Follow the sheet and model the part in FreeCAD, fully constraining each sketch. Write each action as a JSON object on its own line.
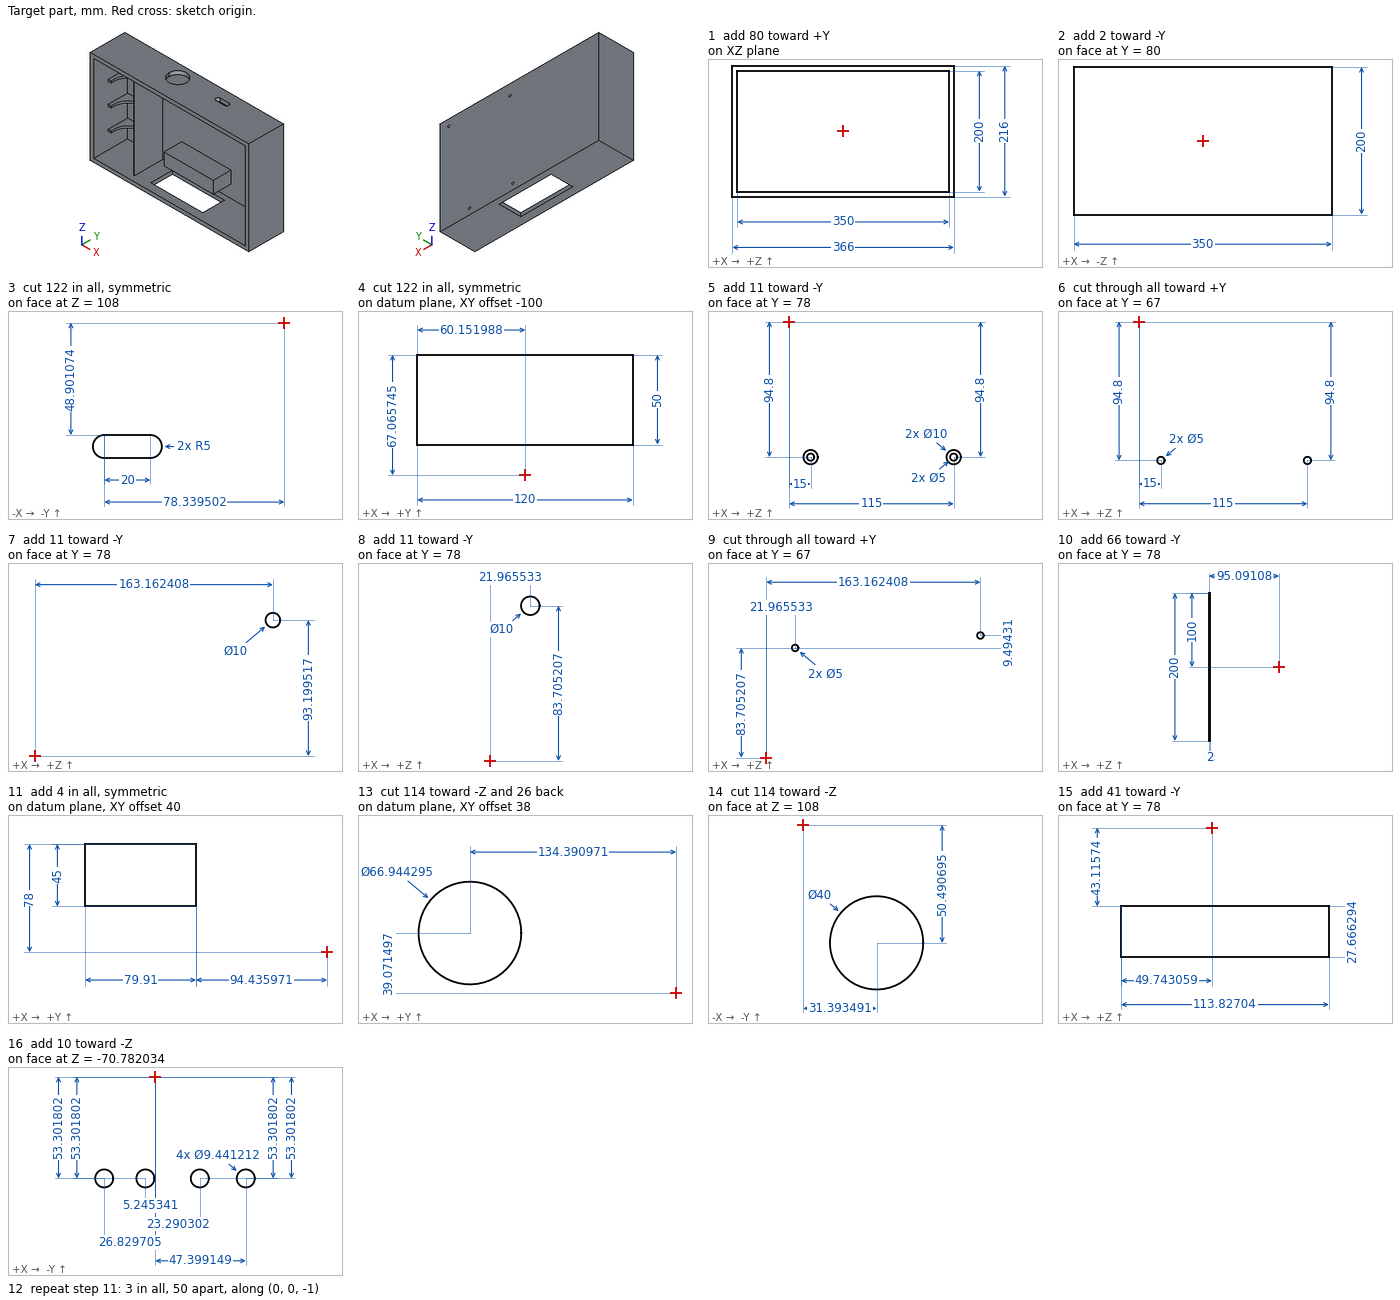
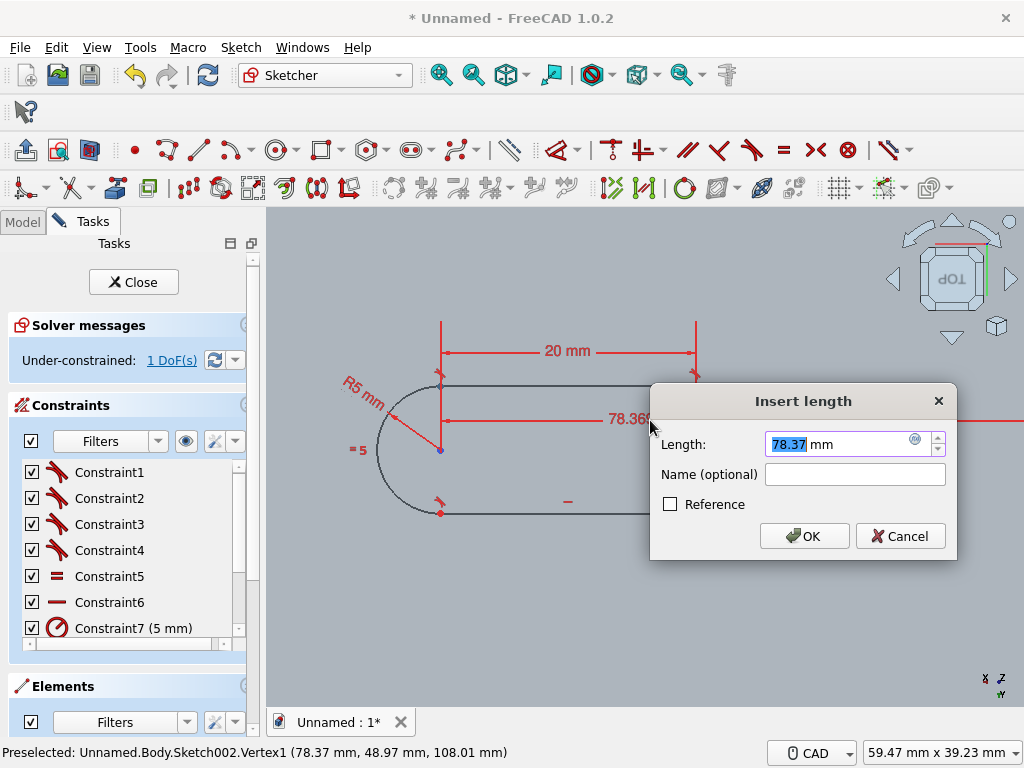
{"action": "type", "text": "78.339502"}
{"action": "key", "text": "Return"}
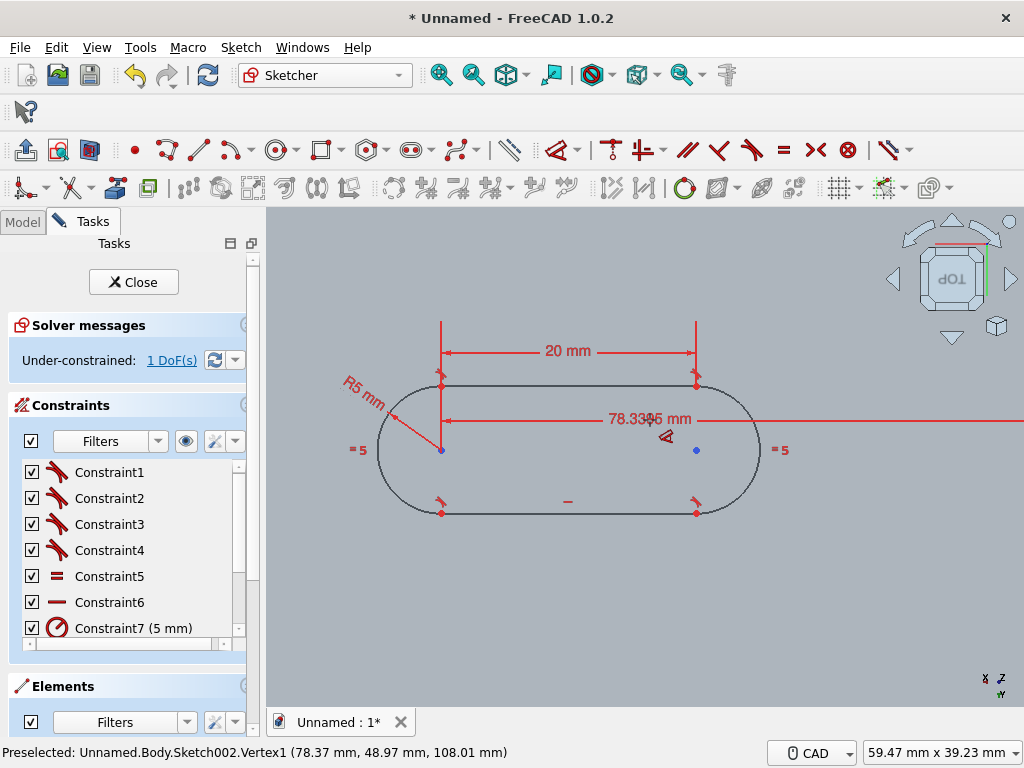
{"action": "left_click", "coordinate": [441, 386]}
{"action": "left_click", "coordinate": [407, 311]}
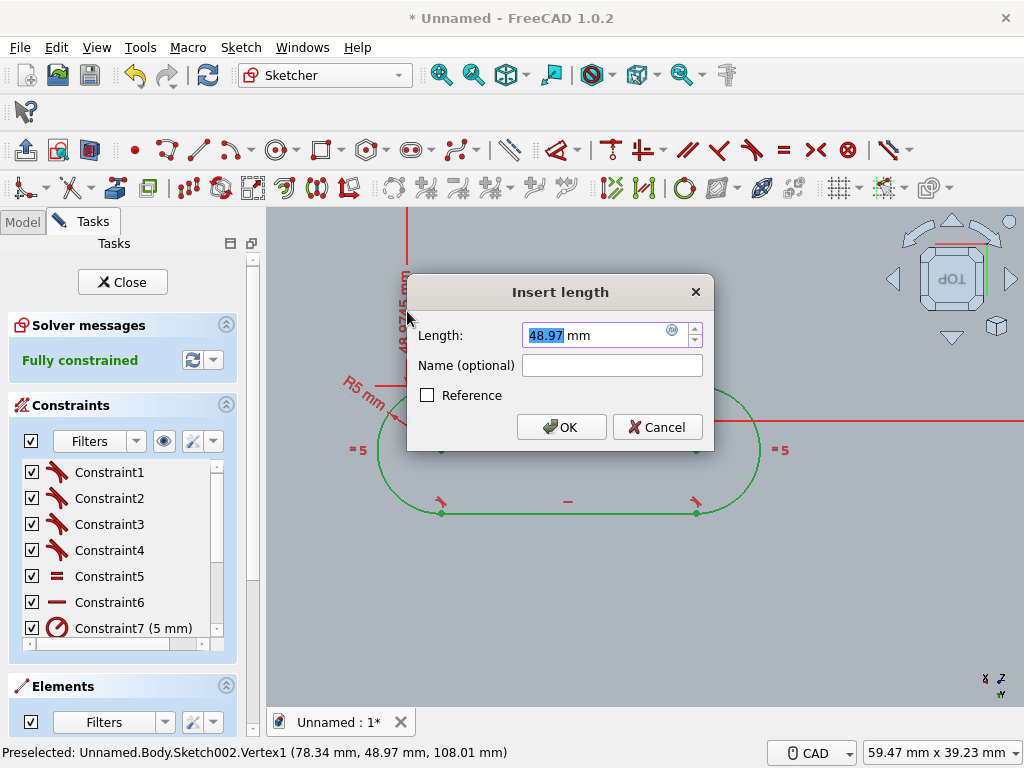
{"action": "type", "text": "48.901074"}
{"action": "key", "text": "Return"}
{"action": "key", "text": "Escape"}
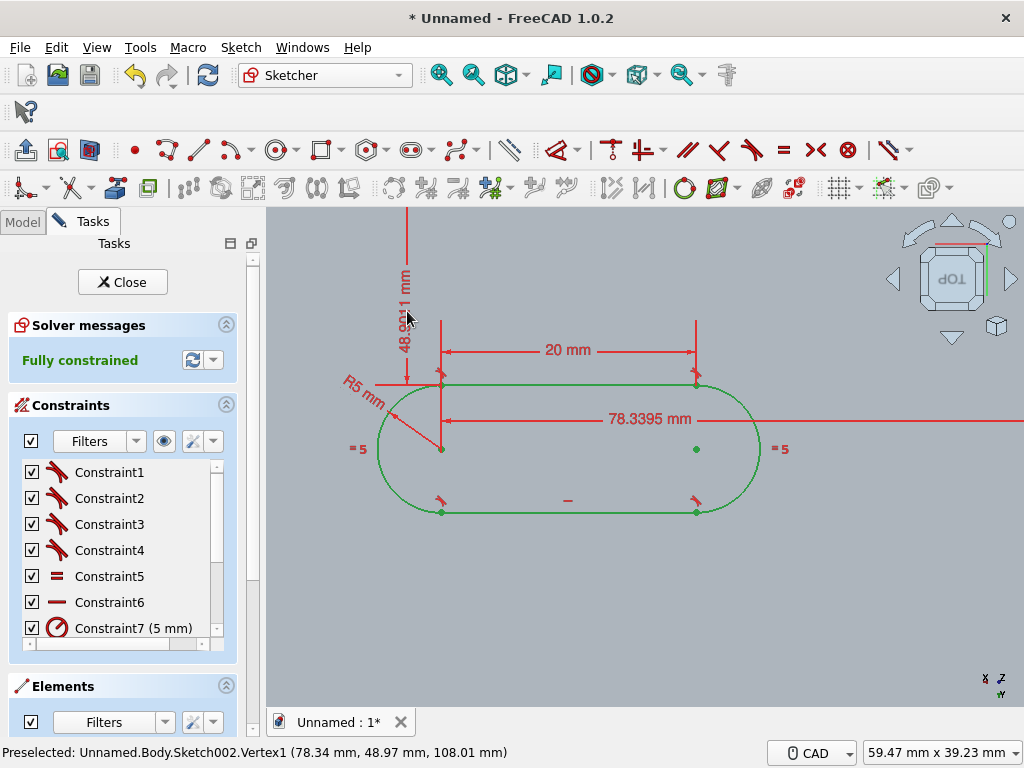
{"action": "left_click", "coordinate": [123, 282]}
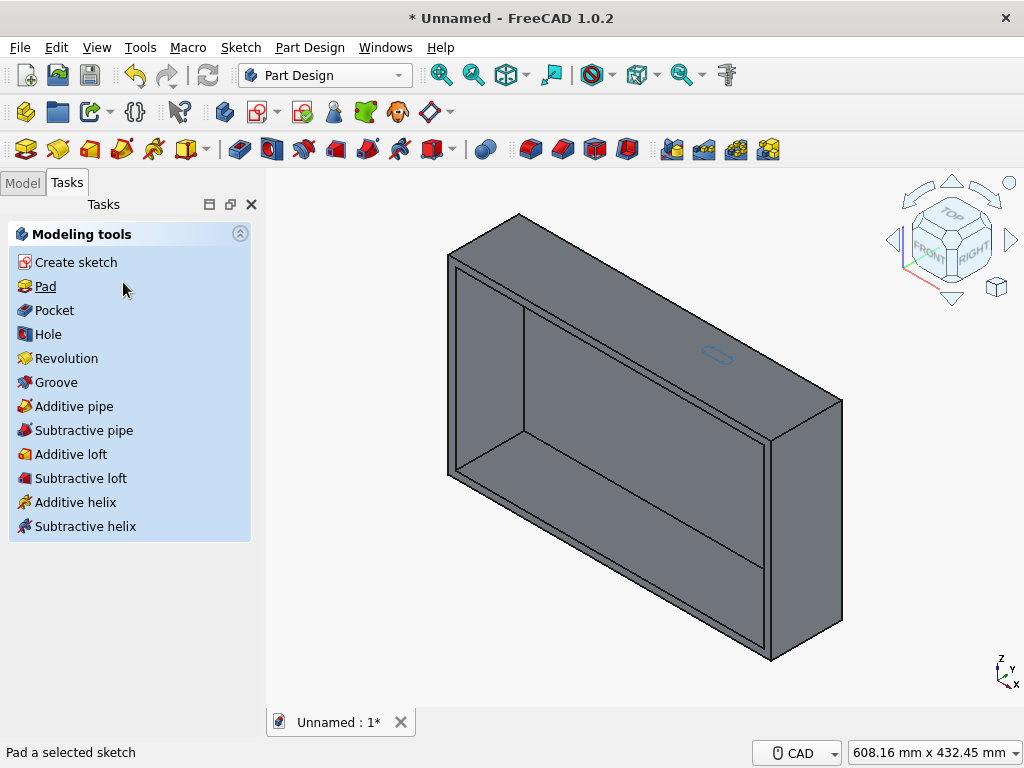
{"action": "left_click", "coordinate": [240, 150]}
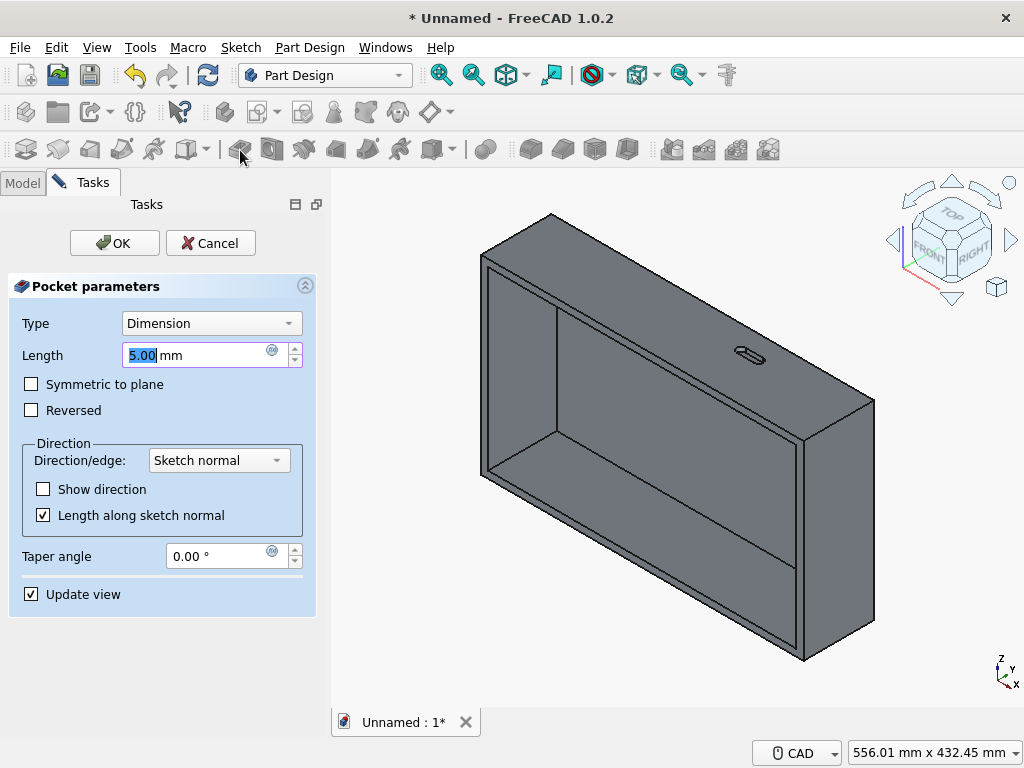
{"action": "type", "text": "122"}
{"action": "key", "text": "Tab"}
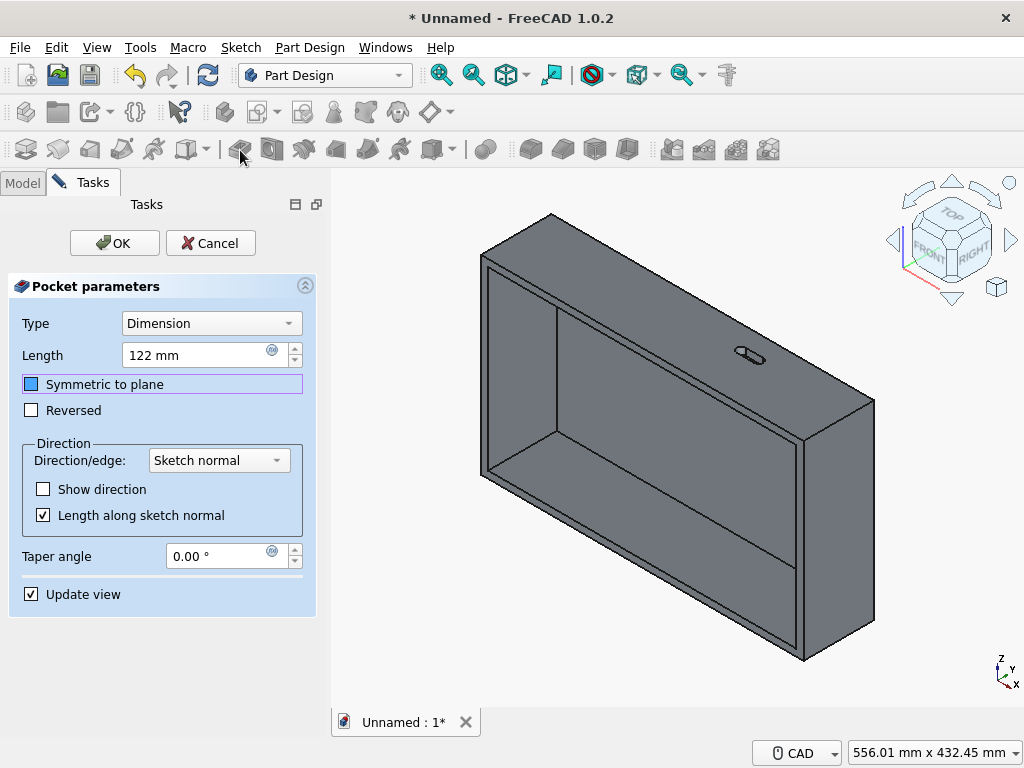
{"action": "left_click", "coordinate": [30, 384]}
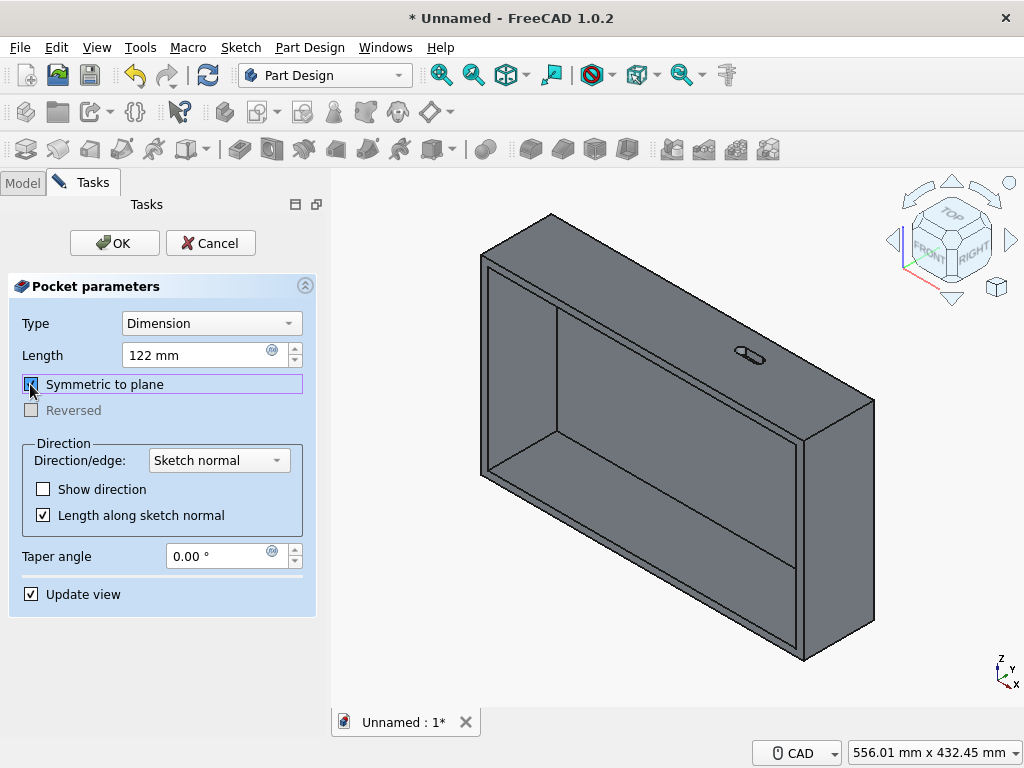
{"action": "left_click", "coordinate": [115, 243]}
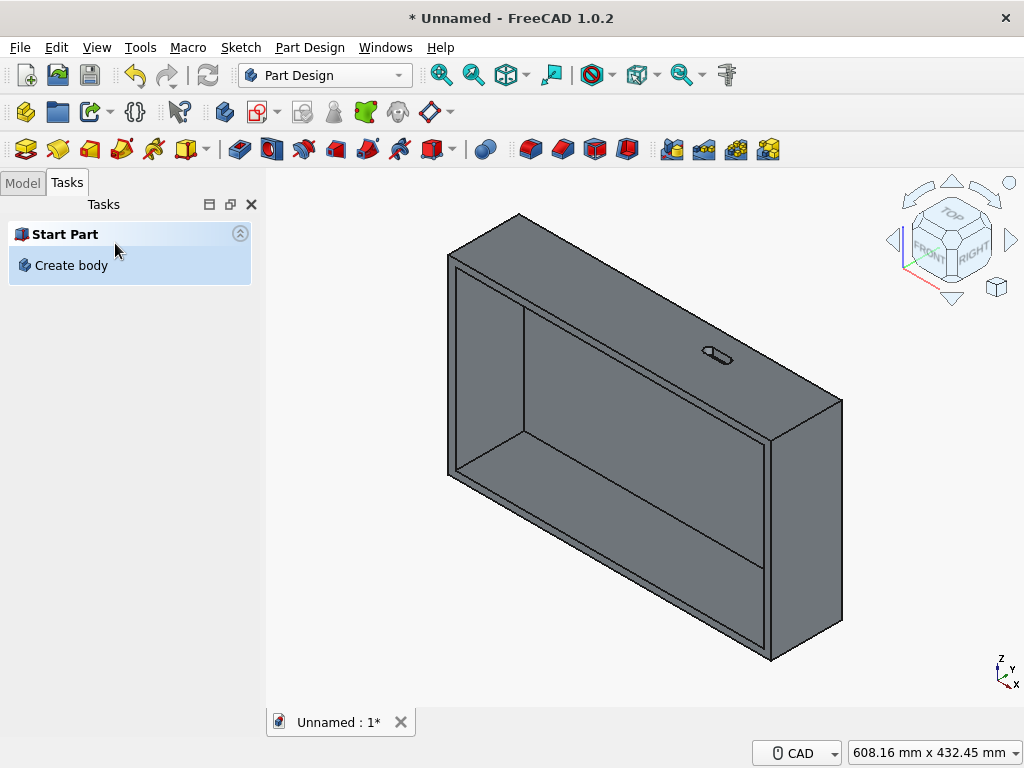
{"action": "left_click", "coordinate": [23, 182]}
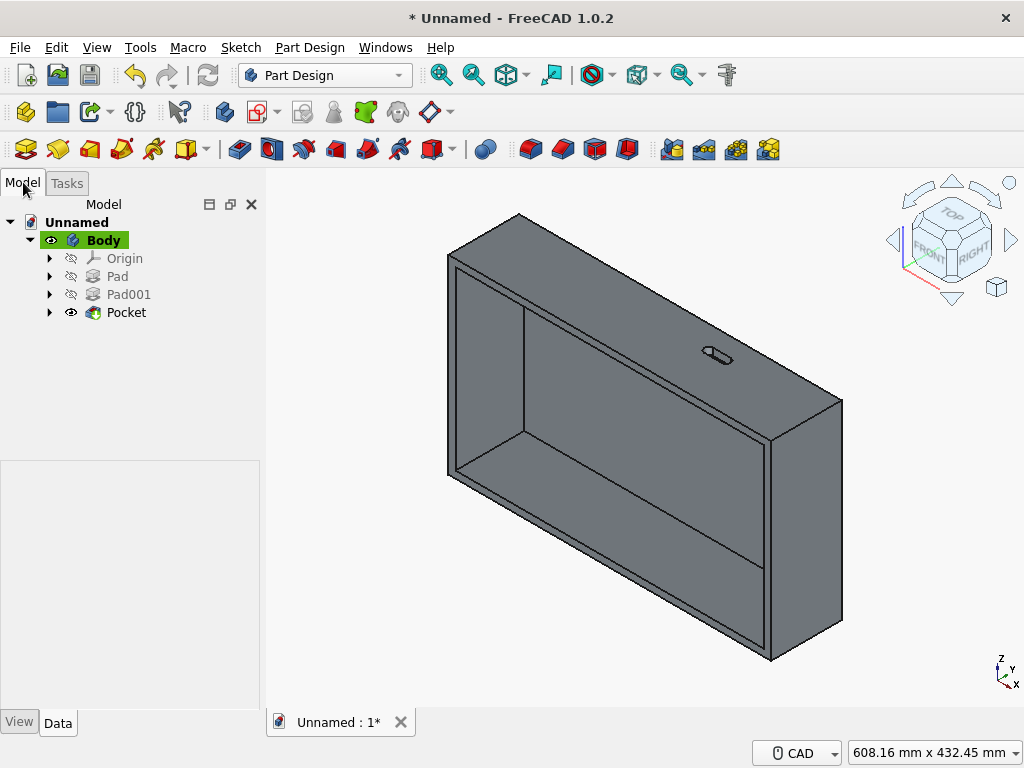
{"action": "left_click", "coordinate": [50, 258]}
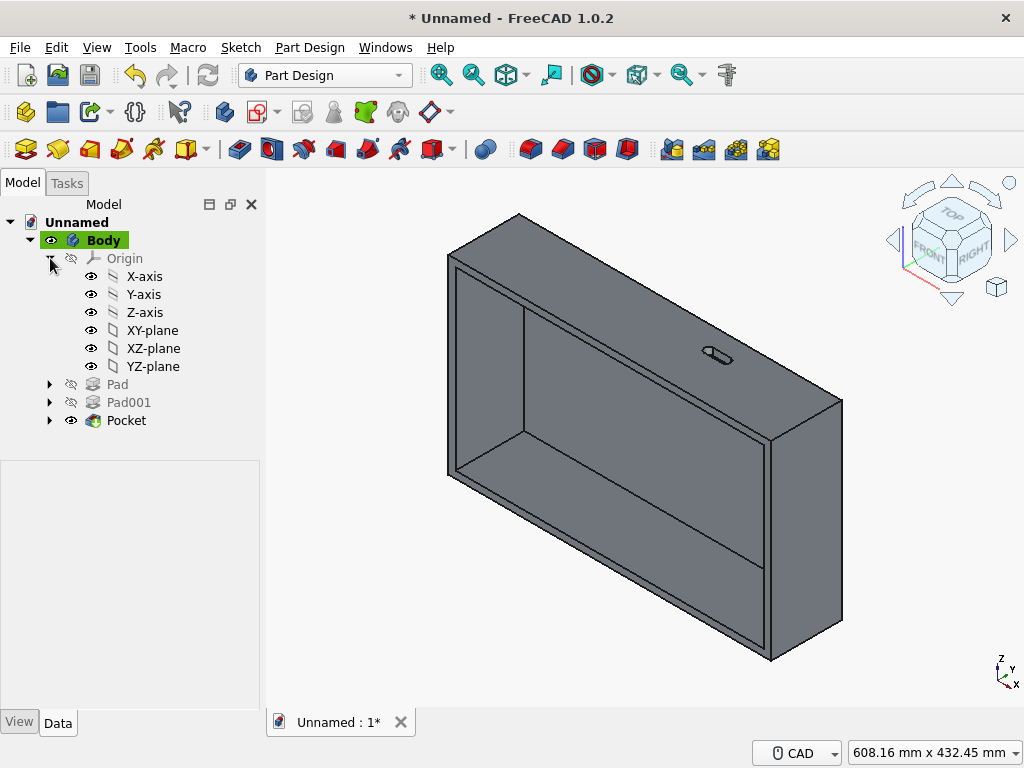
{"action": "left_click", "coordinate": [136, 330]}